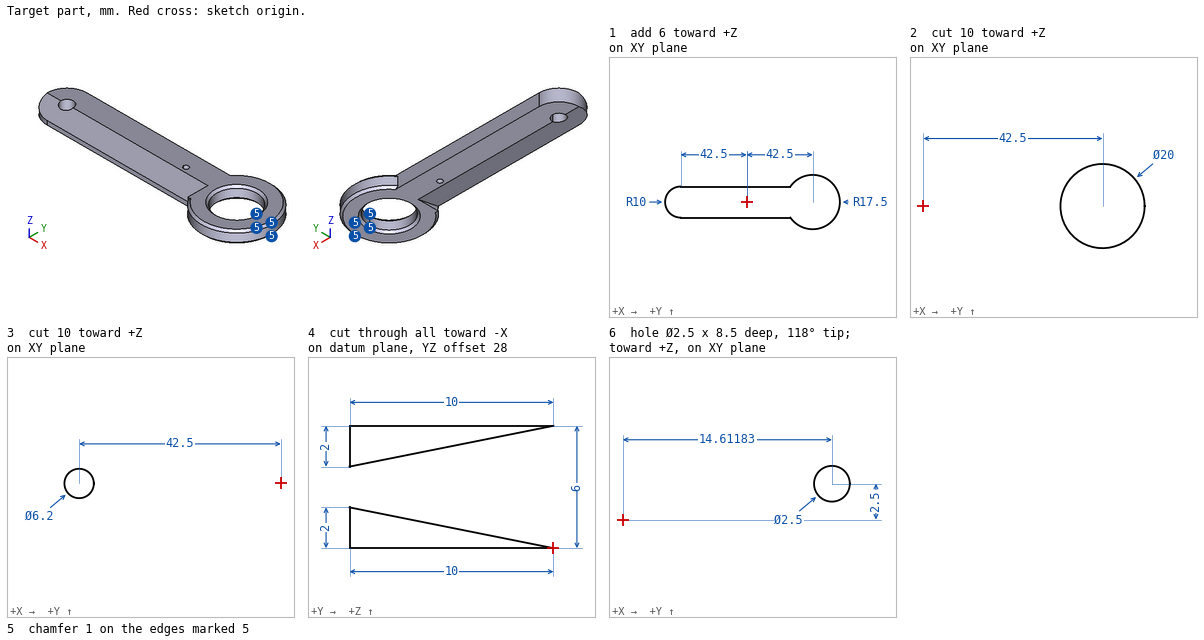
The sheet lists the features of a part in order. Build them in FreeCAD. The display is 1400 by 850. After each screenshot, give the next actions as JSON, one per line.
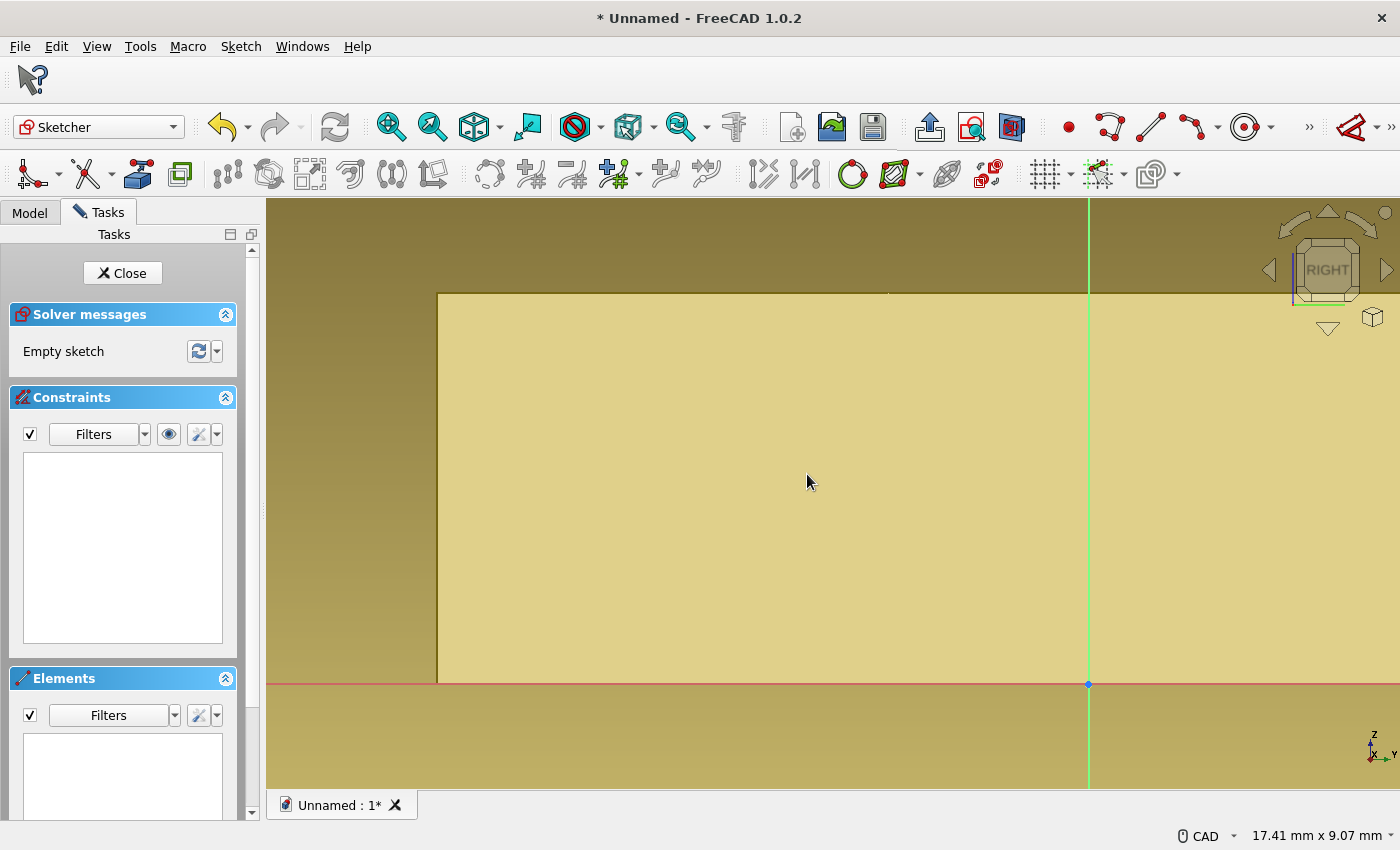
{"action": "left_click", "coordinate": [1110, 128]}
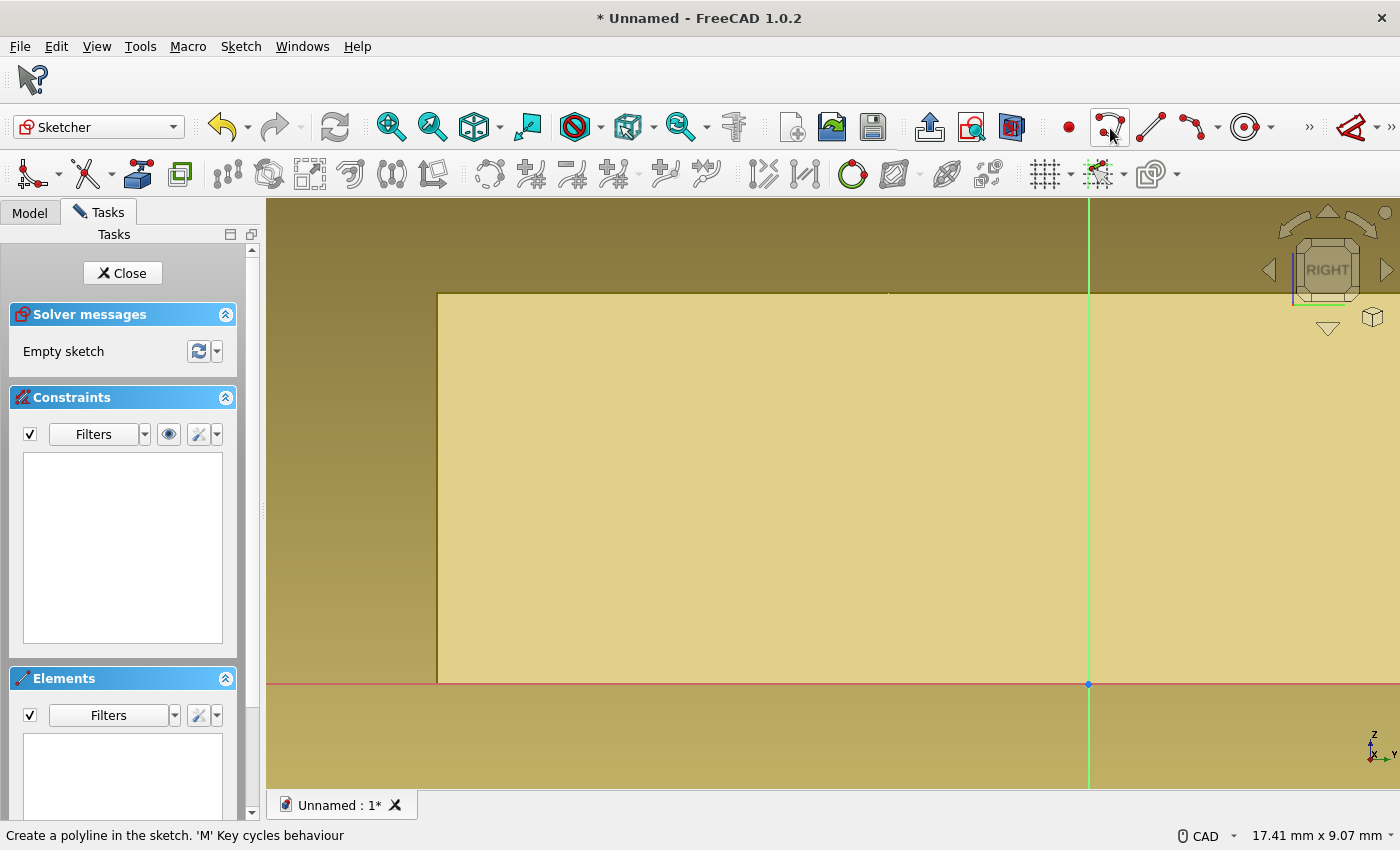
{"action": "left_click", "coordinate": [1089, 293]}
{"action": "left_click", "coordinate": [437, 293]}
{"action": "left_click", "coordinate": [437, 424]}
{"action": "left_click", "coordinate": [1089, 294]}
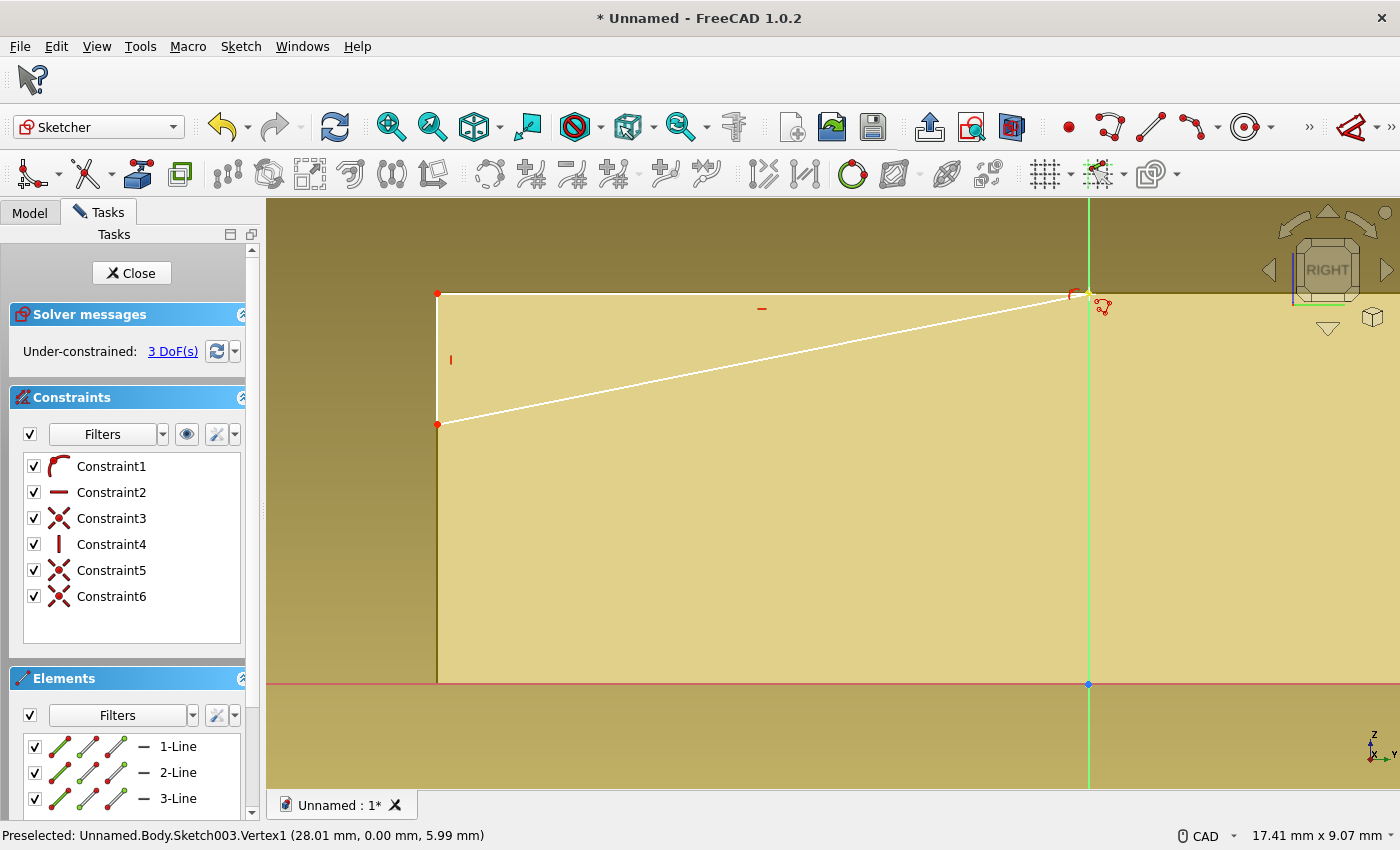
{"action": "left_click", "coordinate": [1089, 684]}
{"action": "left_click", "coordinate": [437, 554]}
{"action": "left_click", "coordinate": [437, 675]}
{"action": "left_click", "coordinate": [1089, 684]}
{"action": "key", "text": "Escape"}
{"action": "key", "text": "Escape"}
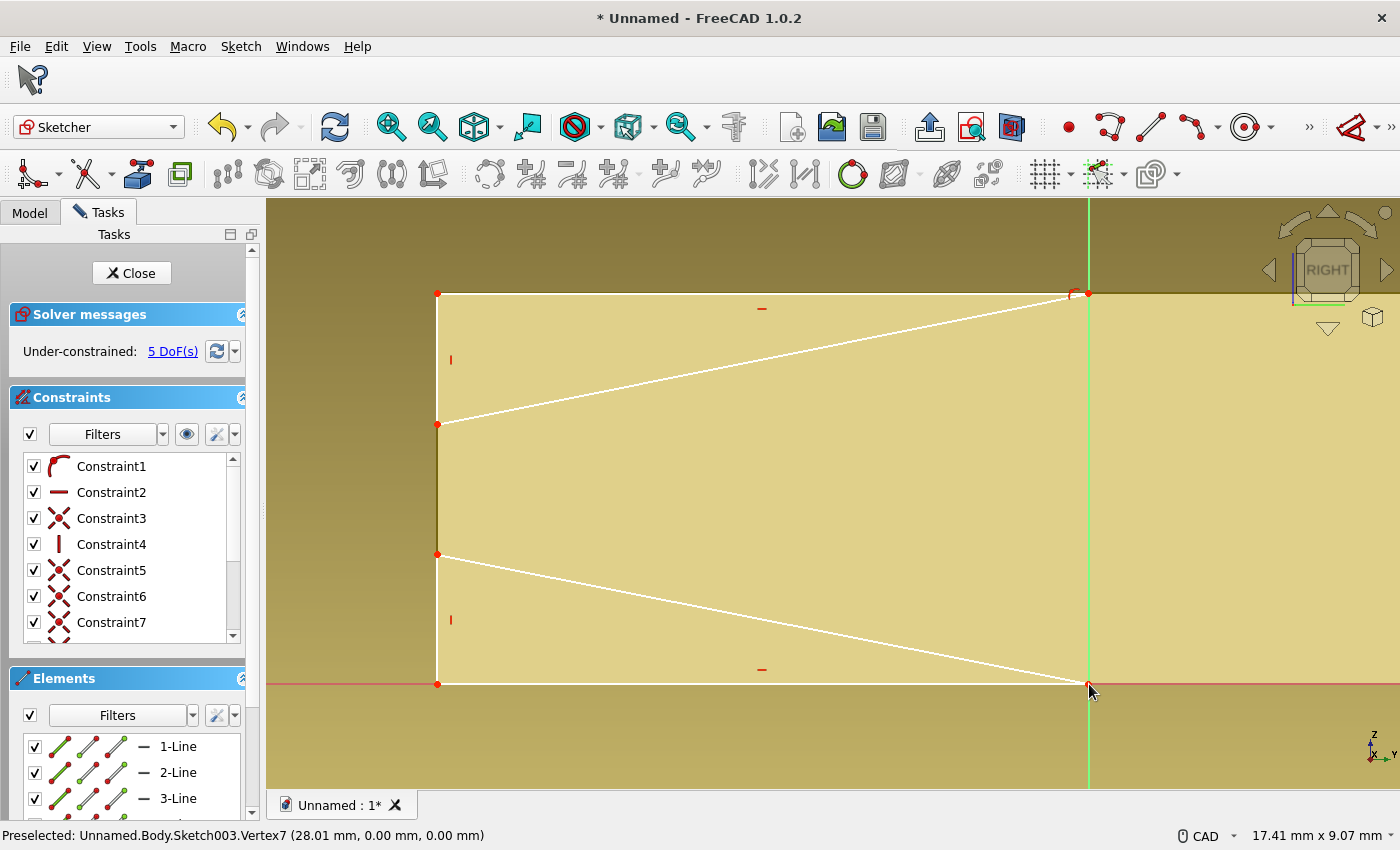
{"action": "key", "text": "d"}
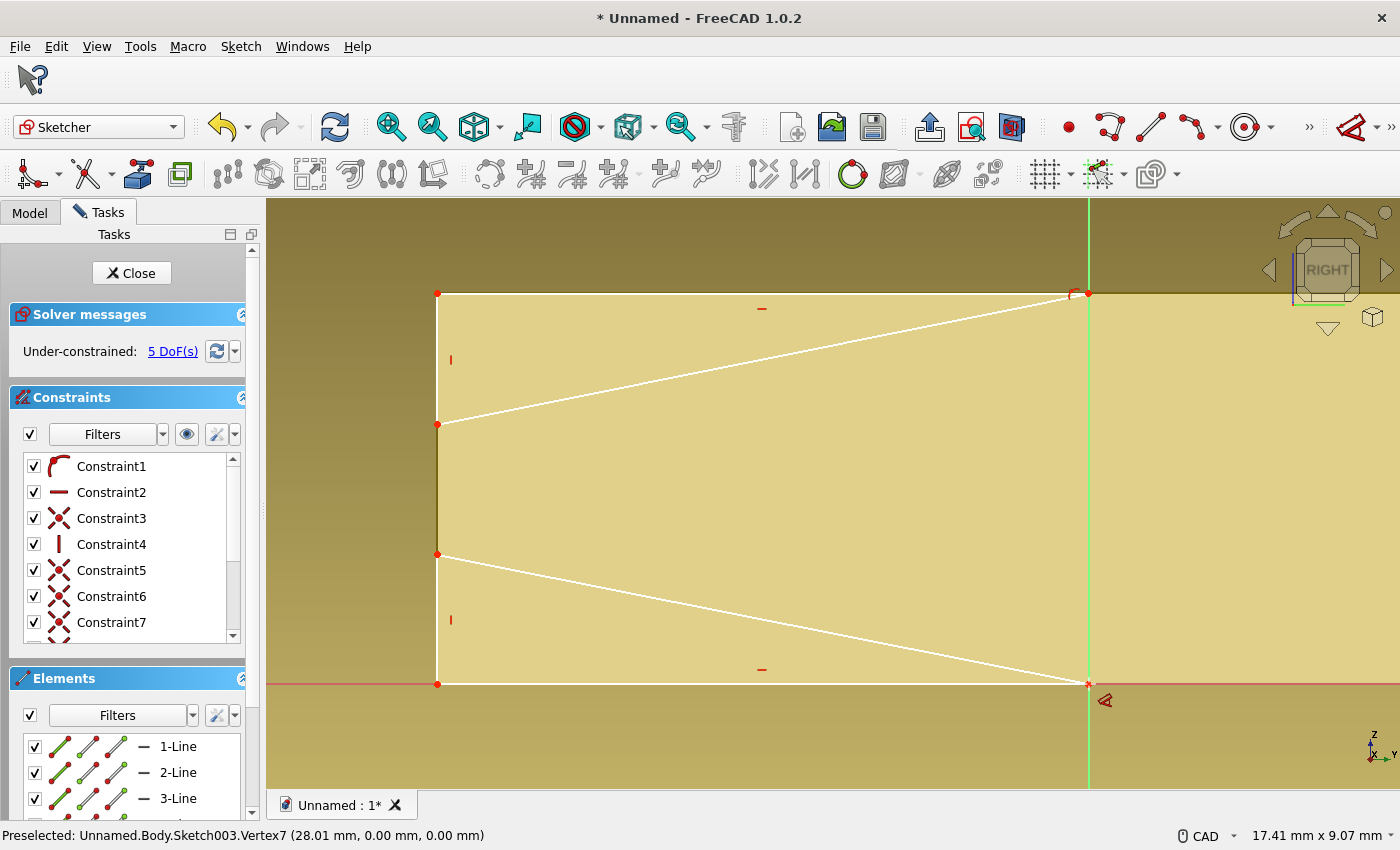
{"action": "left_click", "coordinate": [437, 333]}
{"action": "left_click", "coordinate": [403, 360]}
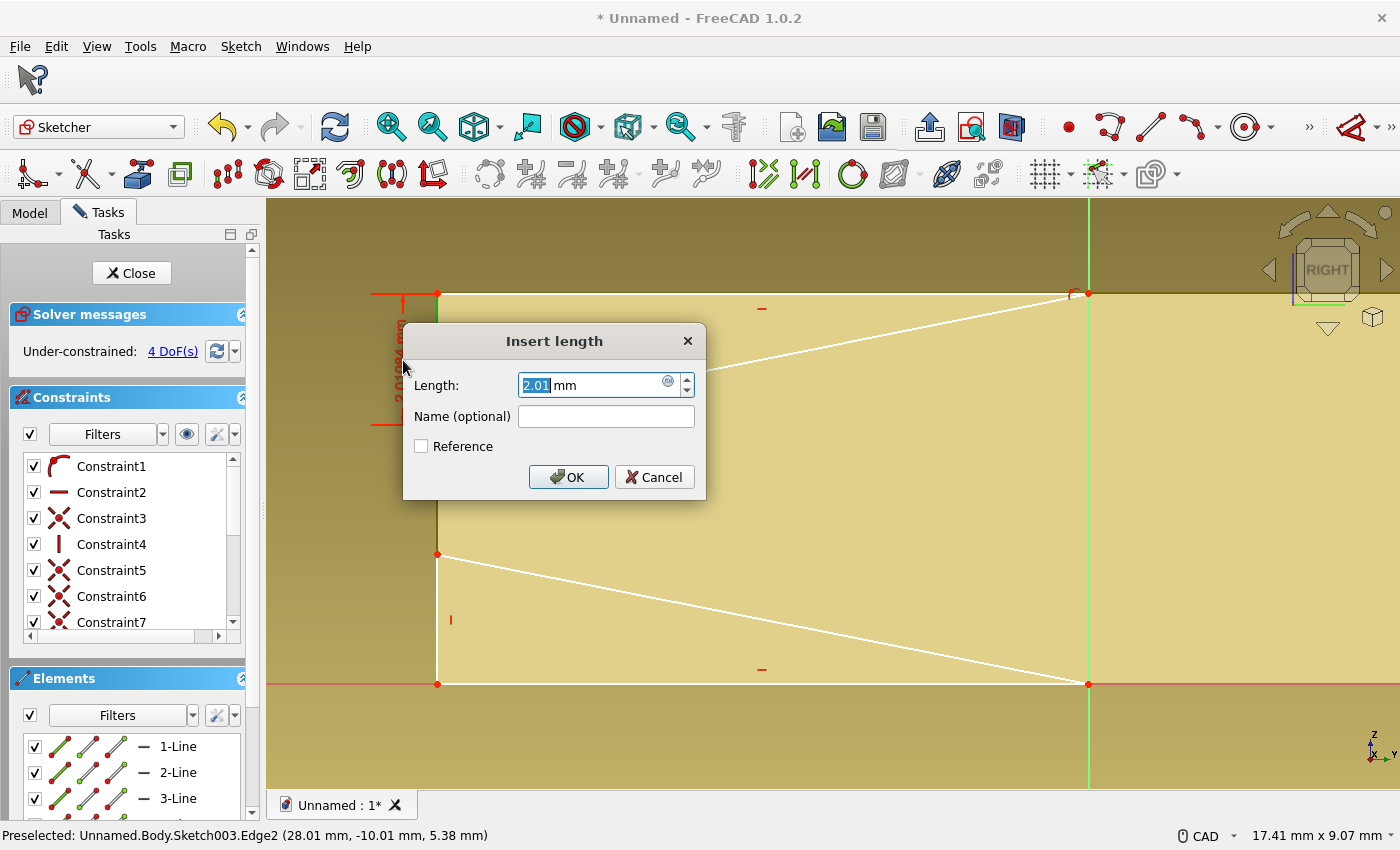
{"action": "type", "text": "2"}
{"action": "key", "text": "Return"}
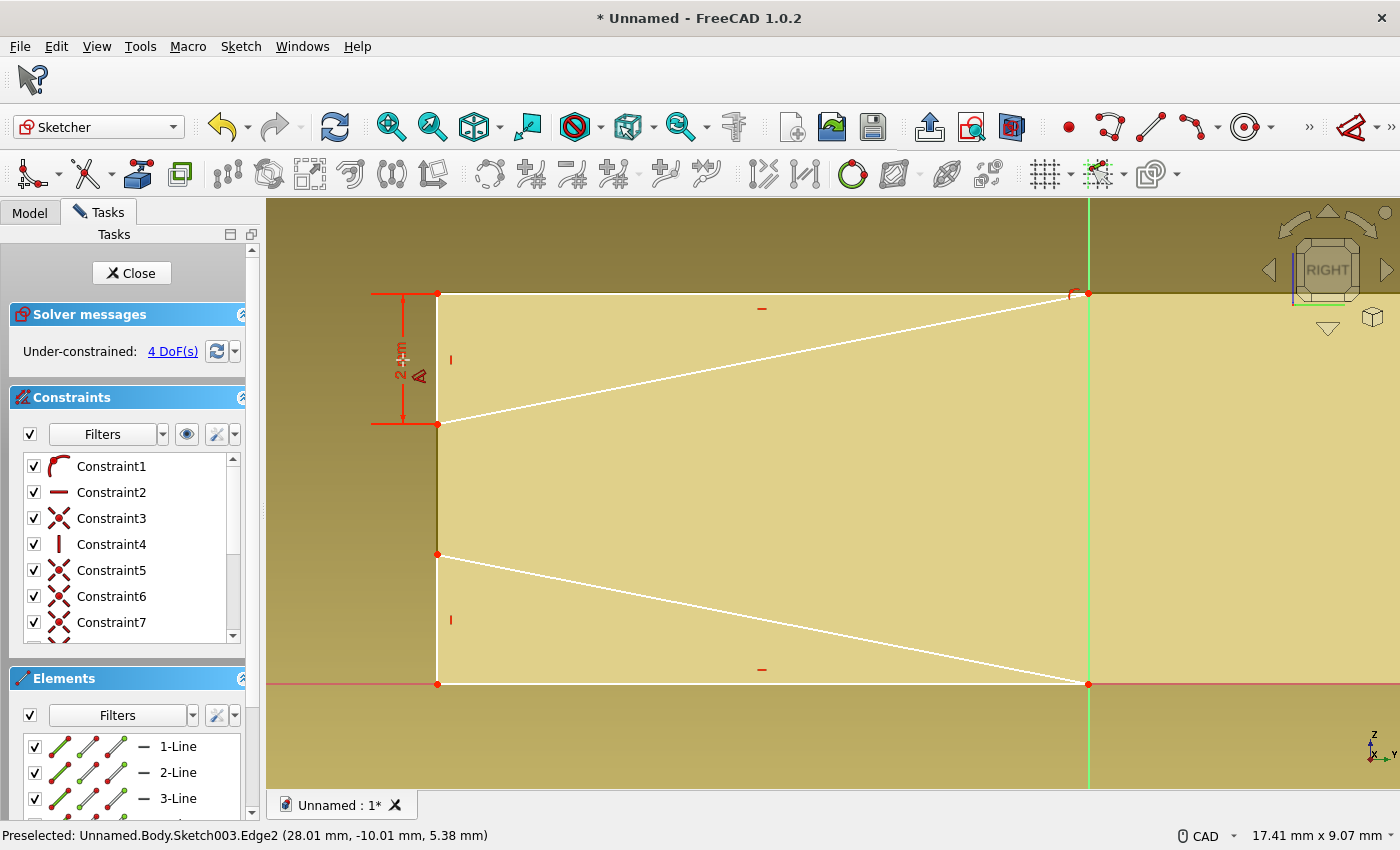
{"action": "left_click", "coordinate": [437, 594]}
{"action": "left_click", "coordinate": [403, 620]}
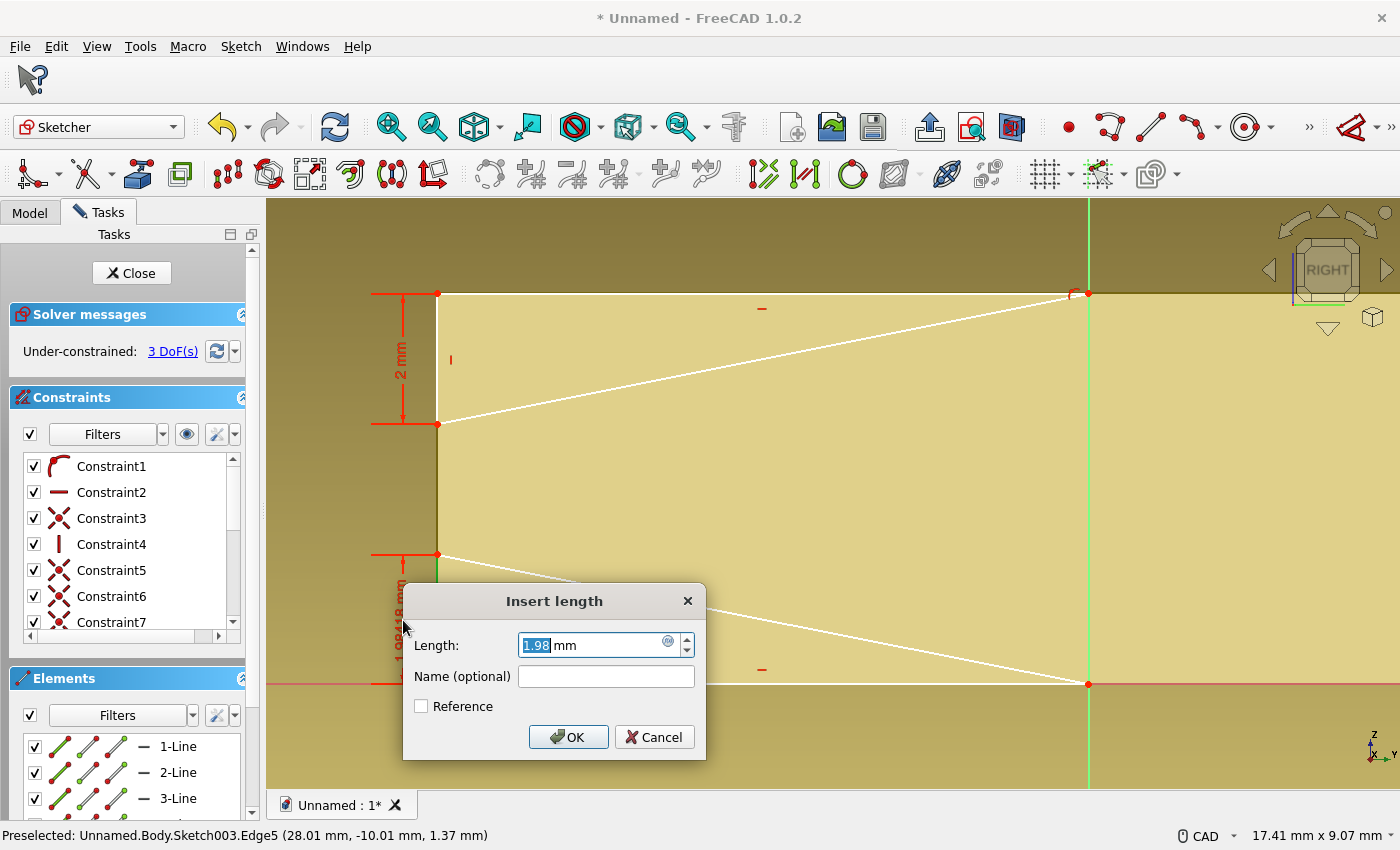
{"action": "type", "text": "2"}
{"action": "key", "text": "Return"}